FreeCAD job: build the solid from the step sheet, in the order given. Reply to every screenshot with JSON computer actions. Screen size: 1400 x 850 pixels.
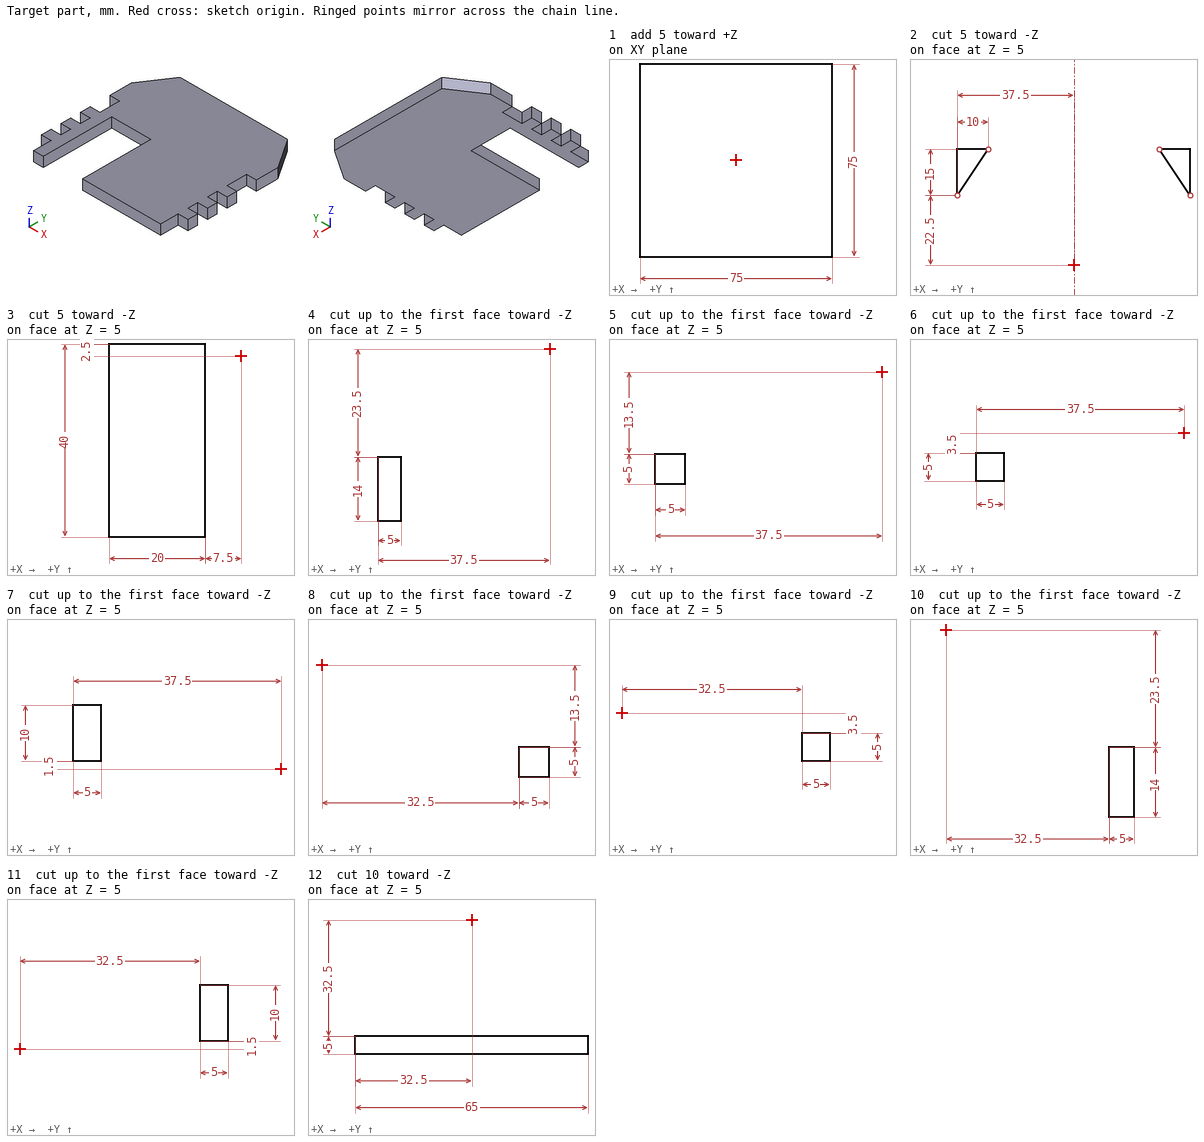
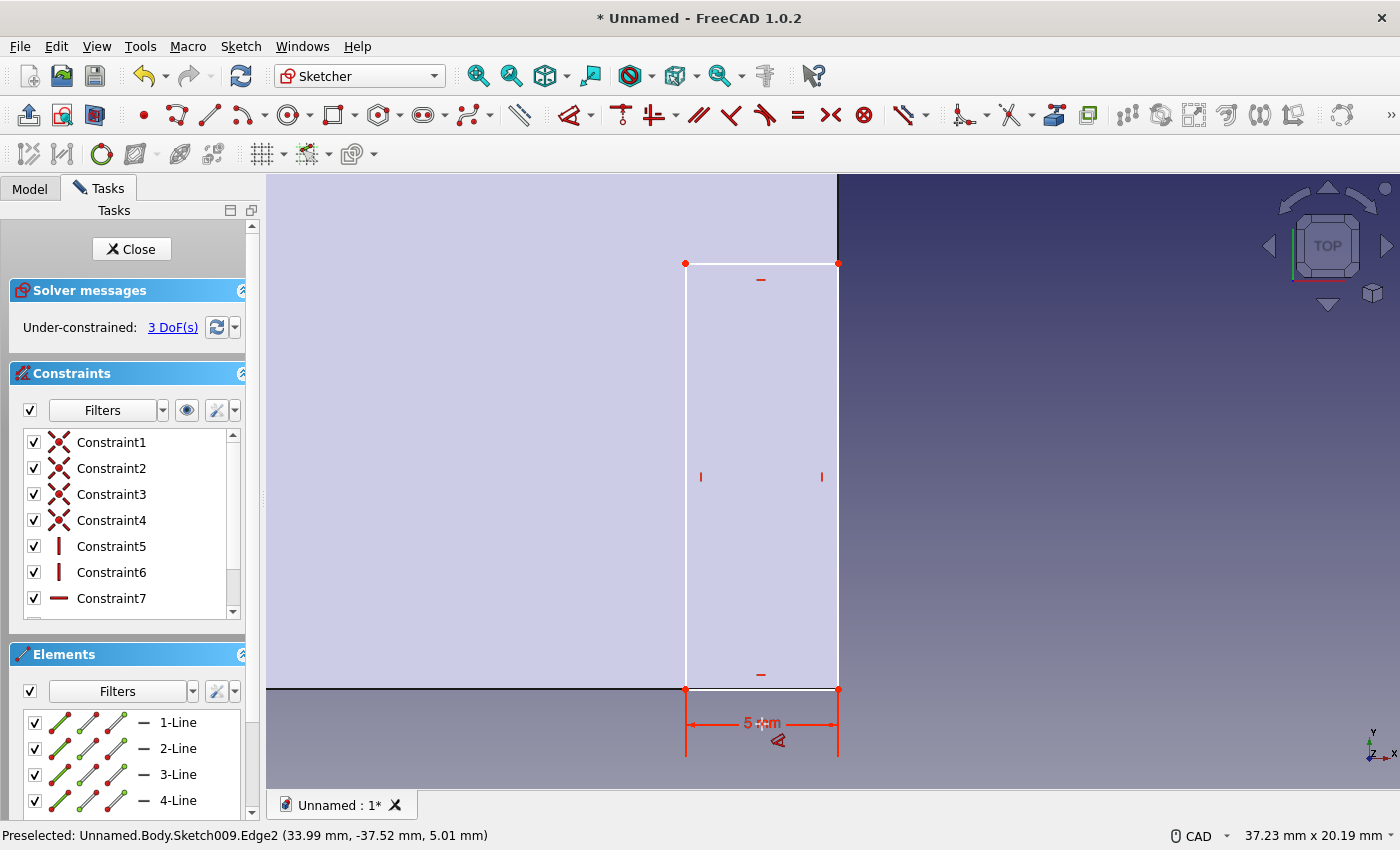
{"action": "left_click", "coordinate": [686, 392]}
{"action": "left_click", "coordinate": [652, 477]}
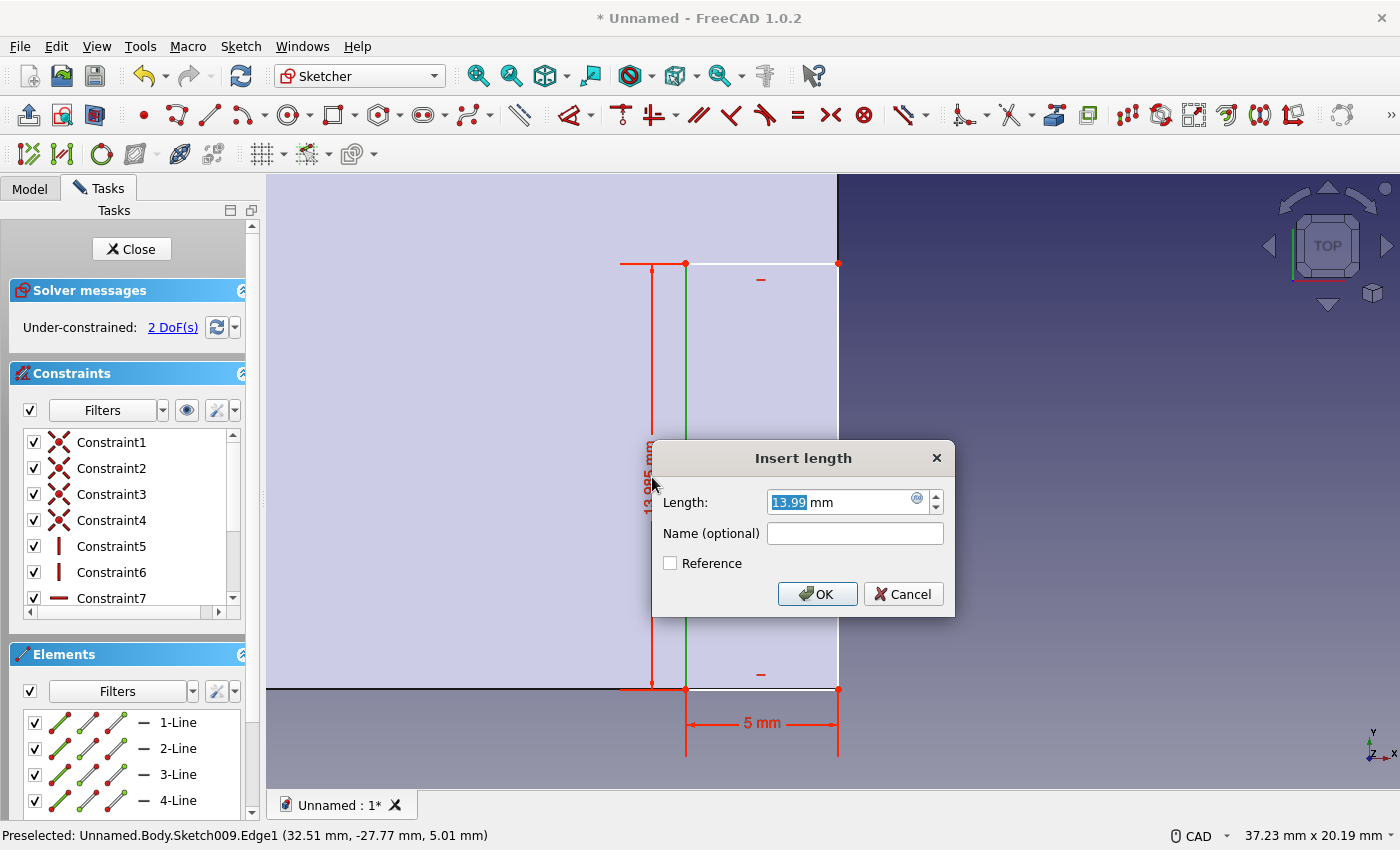
{"action": "type", "text": "14"}
{"action": "key", "text": "Return"}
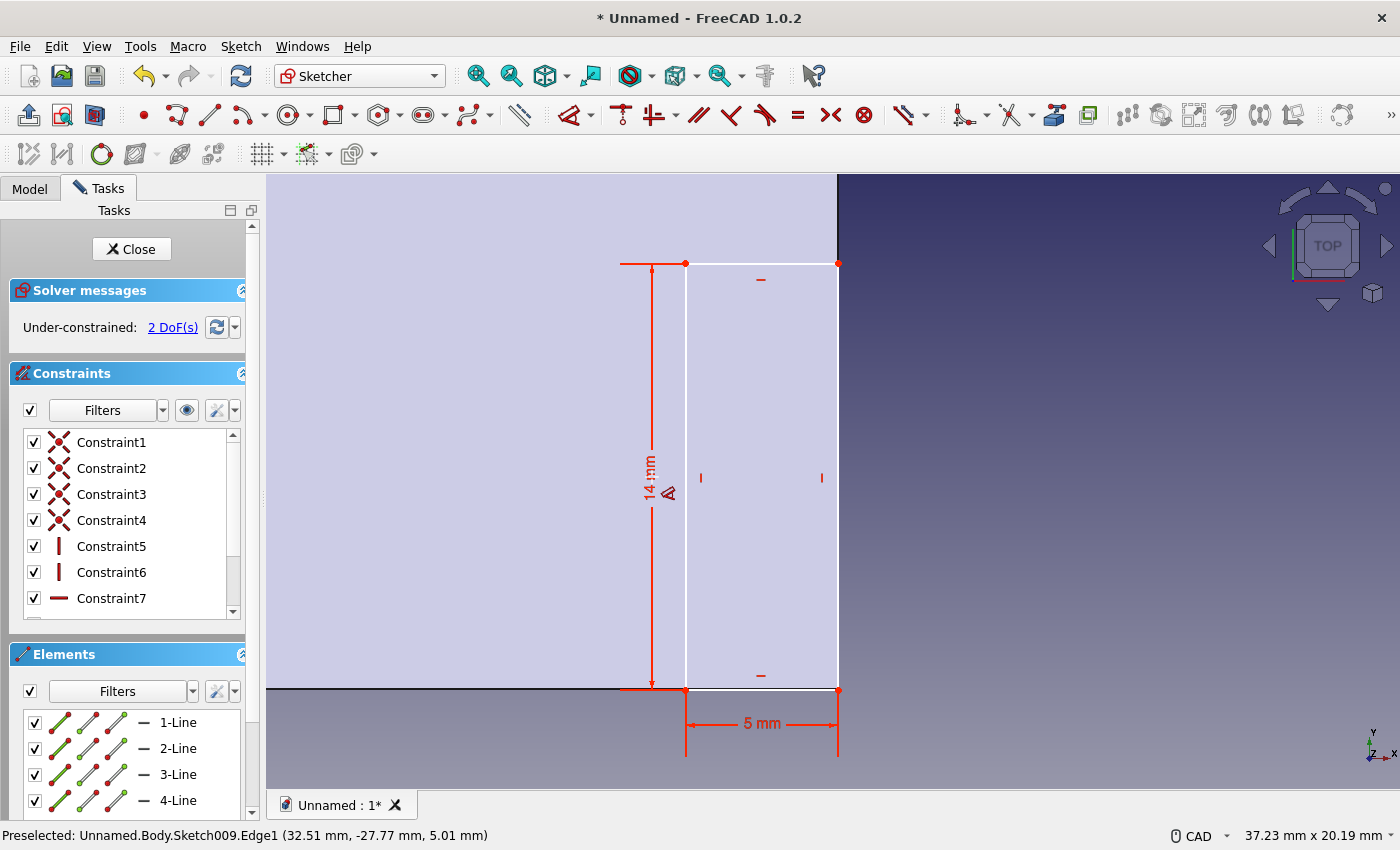
{"action": "left_click", "coordinate": [686, 264]}
{"action": "left_click", "coordinate": [490, 298]}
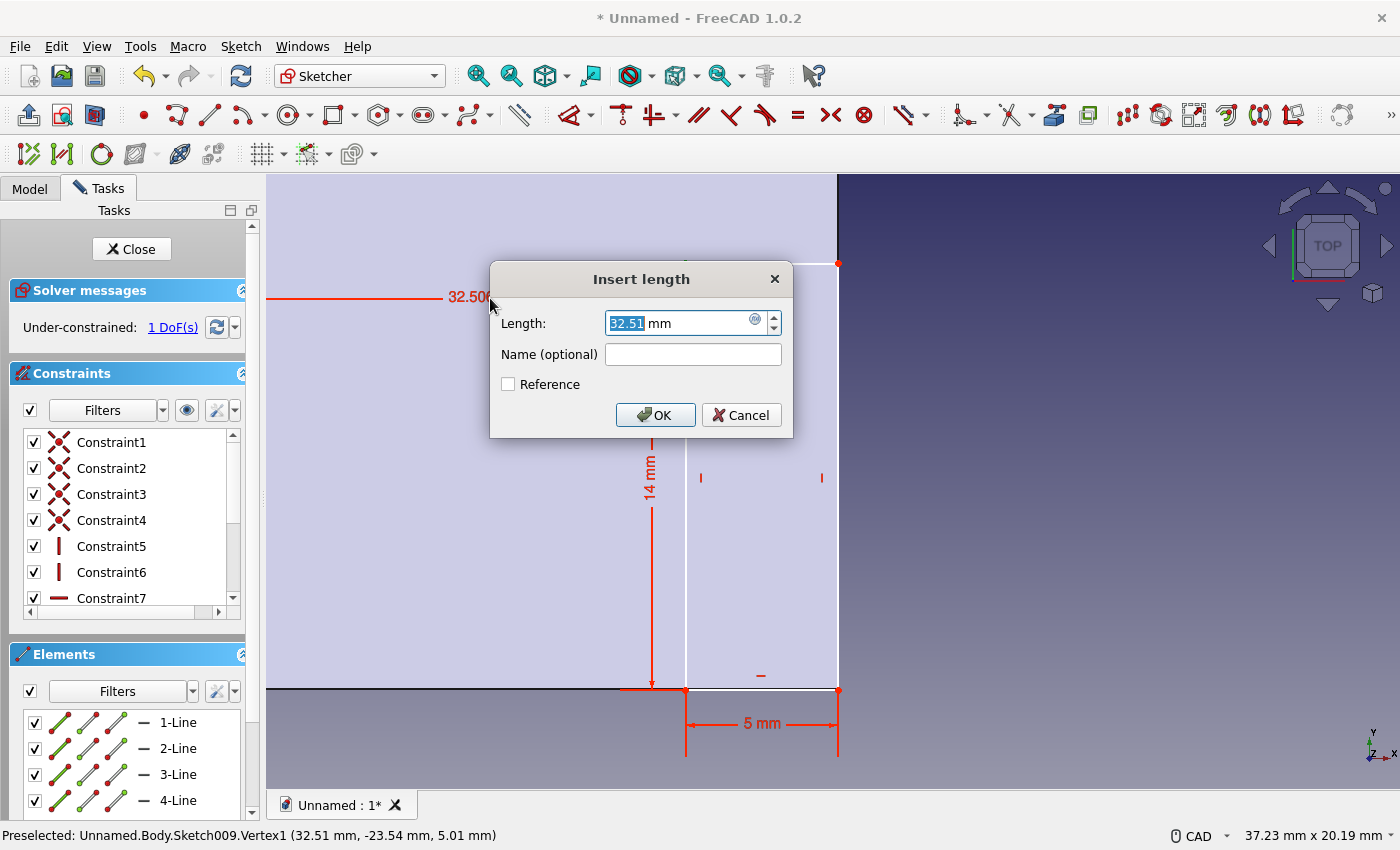
{"action": "type", "text": "32.5"}
{"action": "key", "text": "Return"}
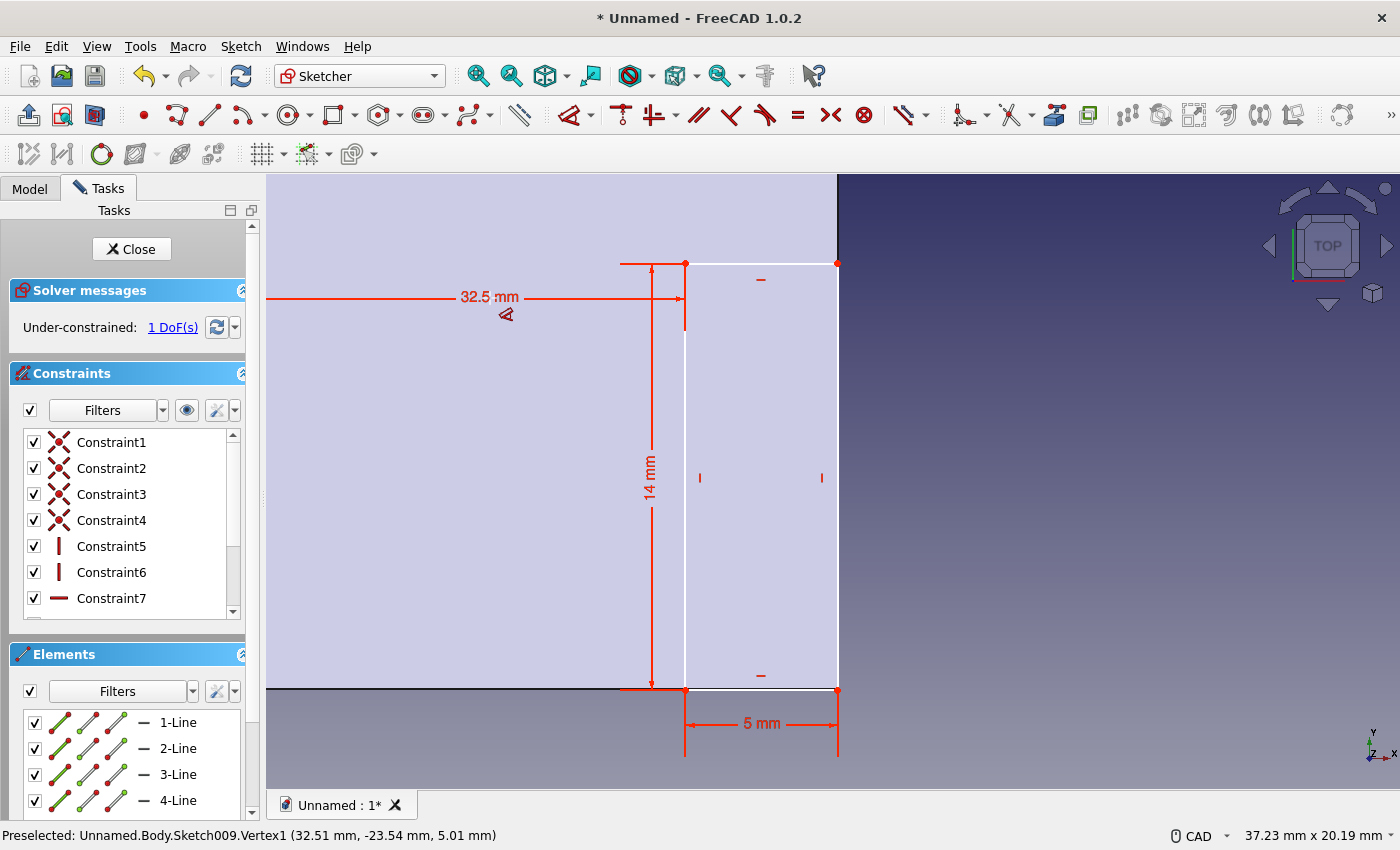
{"action": "left_click", "coordinate": [685, 264]}
{"action": "left_click", "coordinate": [719, 233]}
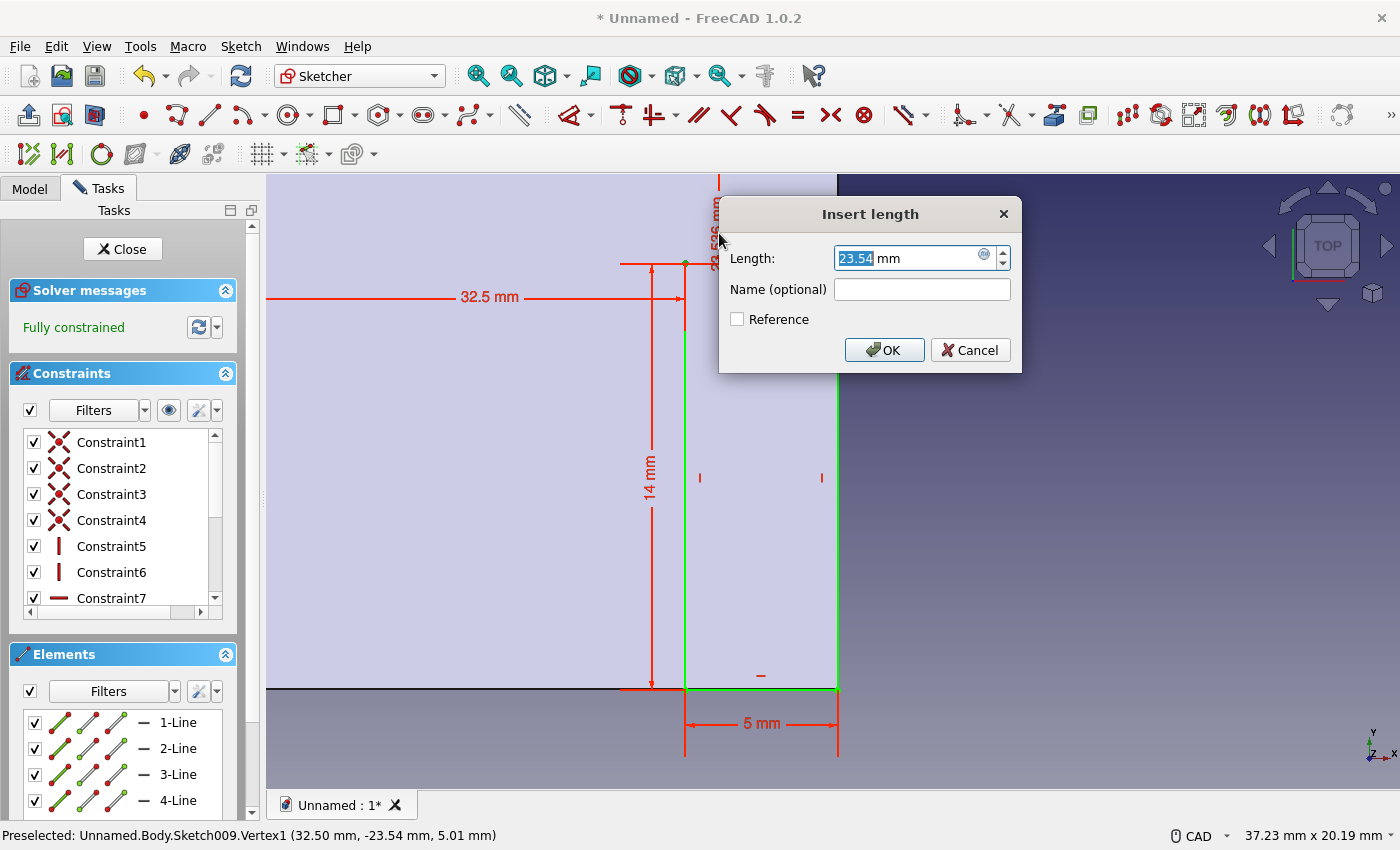
{"action": "type", "text": "23.5"}
{"action": "key", "text": "Return"}
{"action": "key", "text": "Escape"}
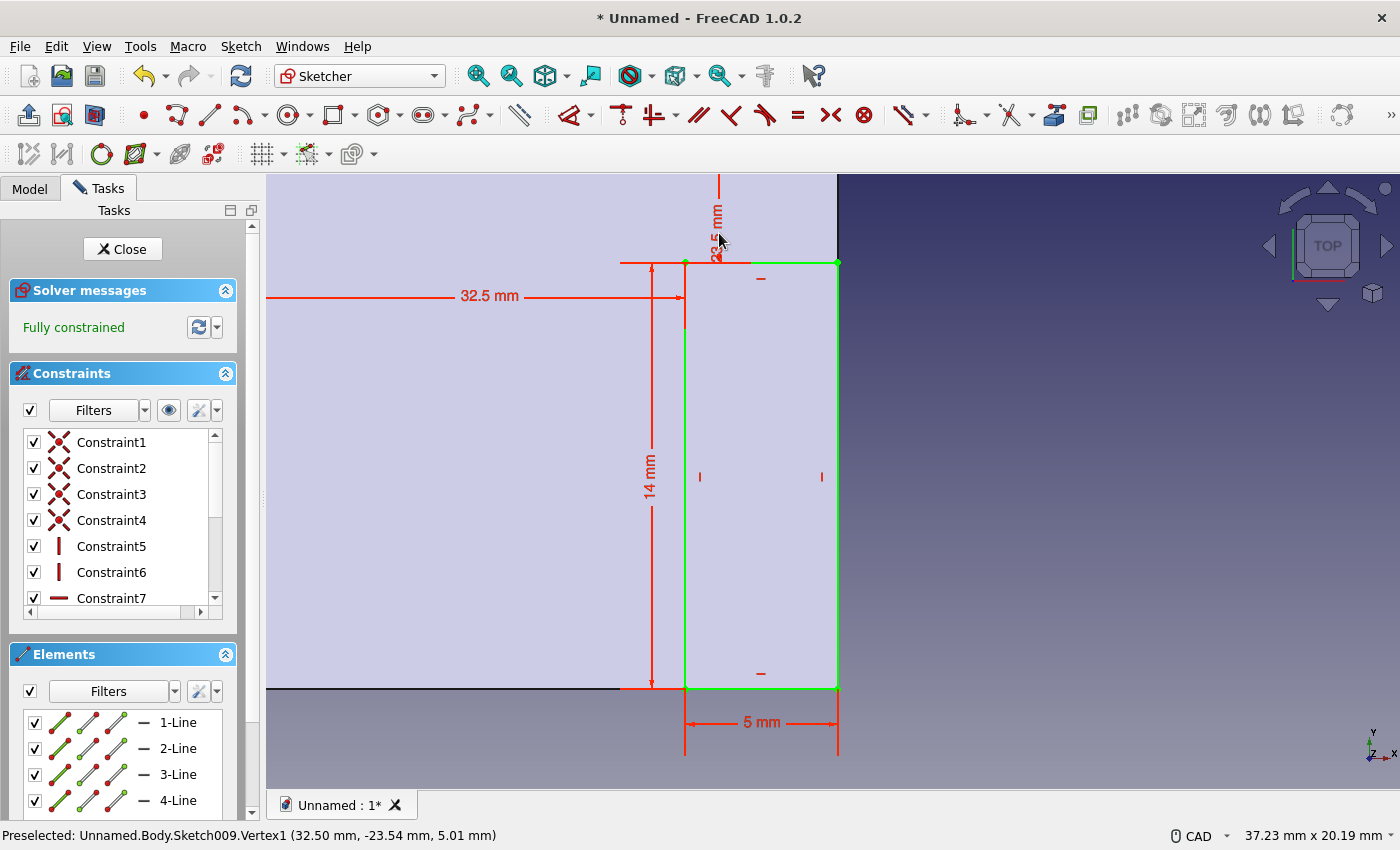
{"action": "left_click", "coordinate": [123, 249]}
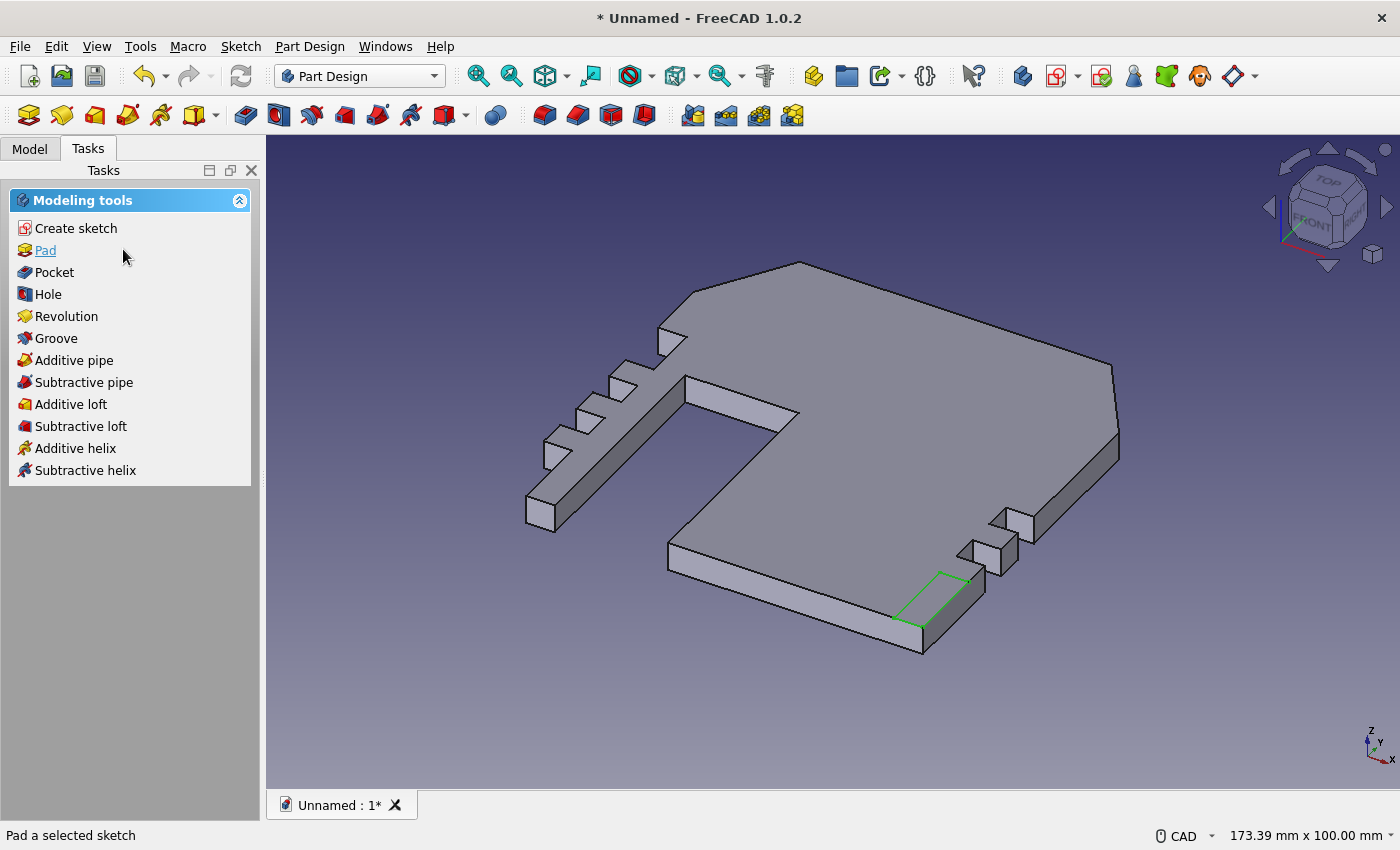
{"action": "left_click", "coordinate": [246, 116]}